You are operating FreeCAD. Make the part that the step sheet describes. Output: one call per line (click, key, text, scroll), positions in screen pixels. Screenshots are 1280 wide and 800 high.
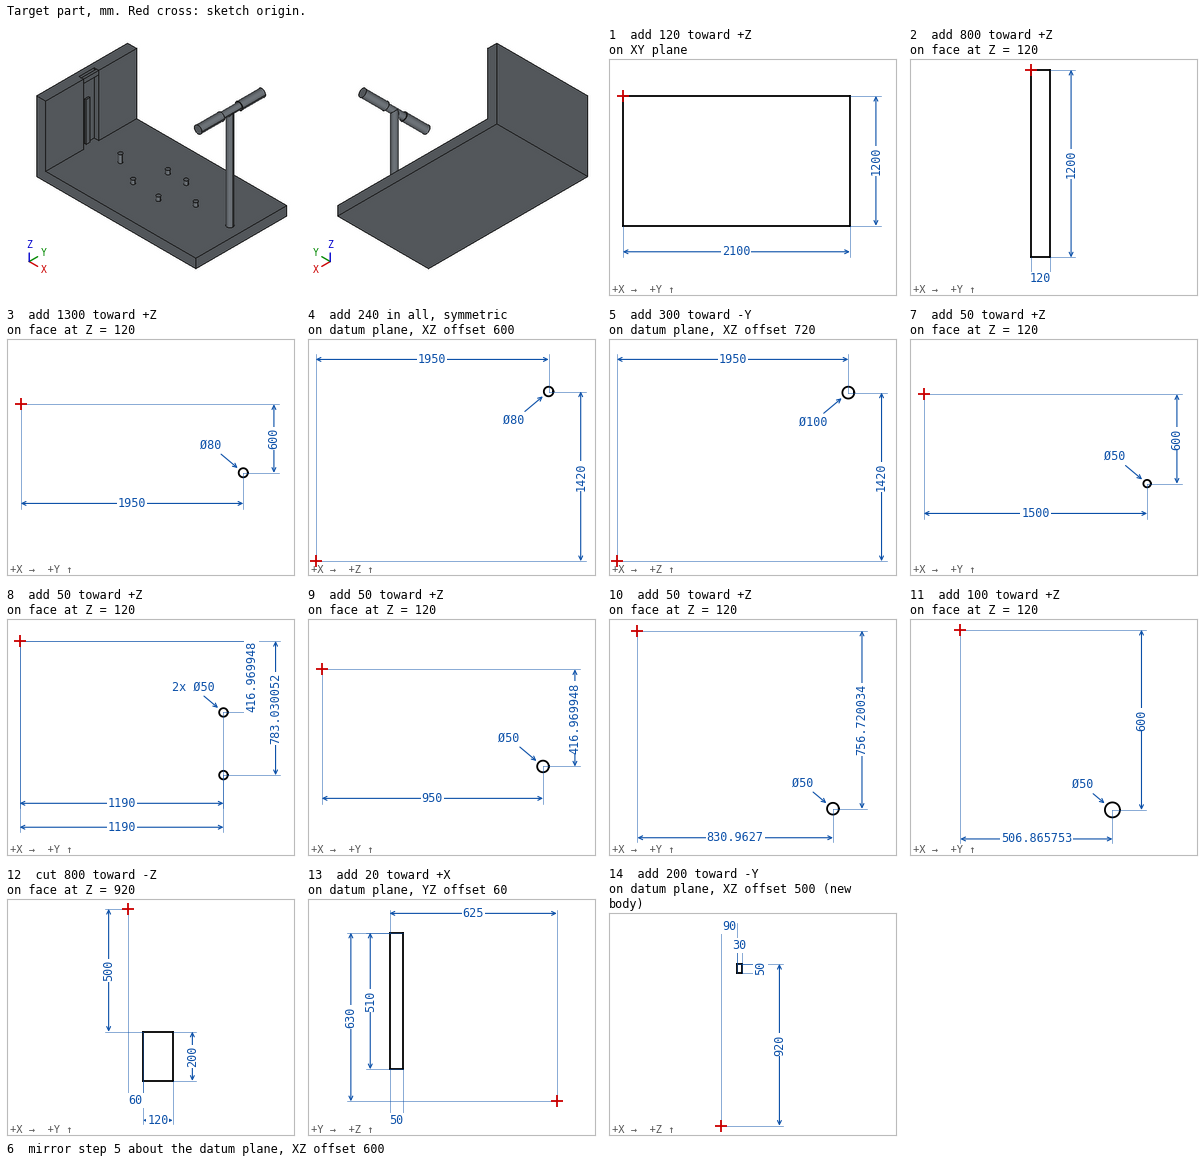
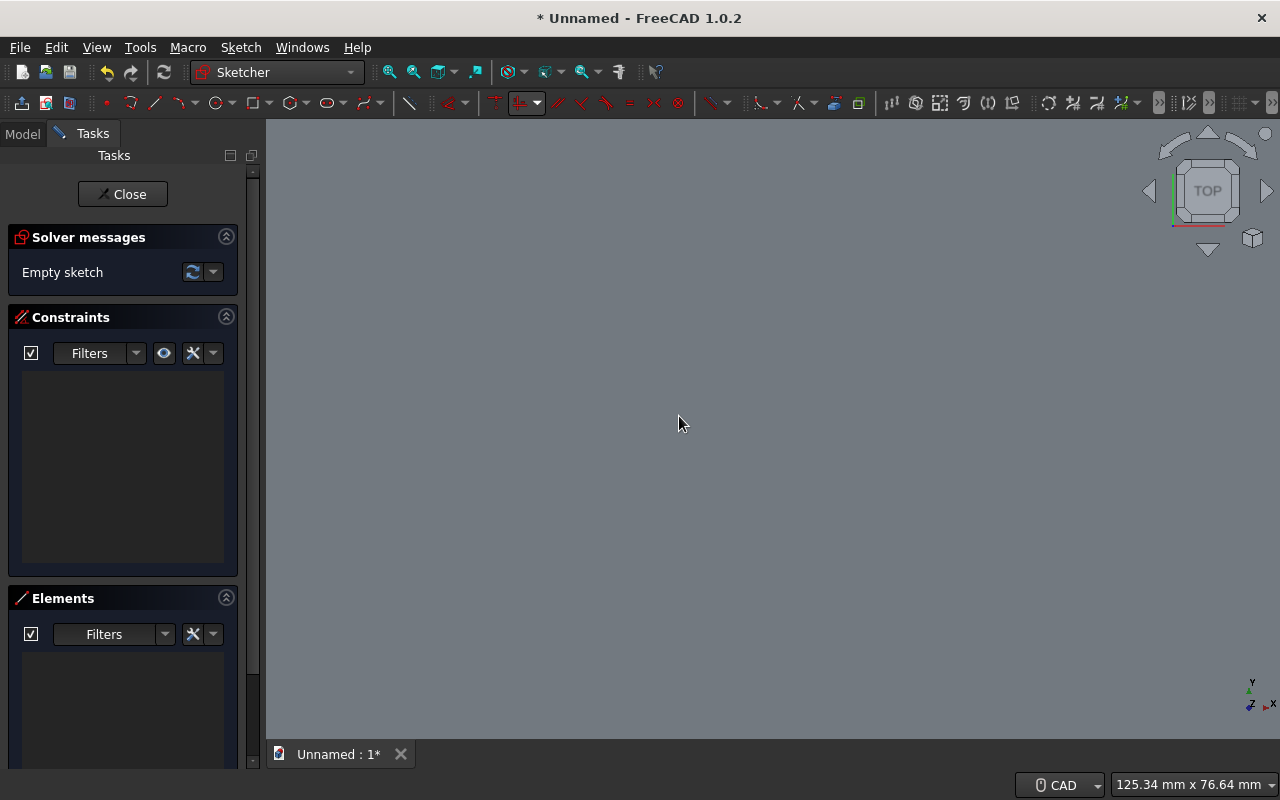
key(g)
key(c)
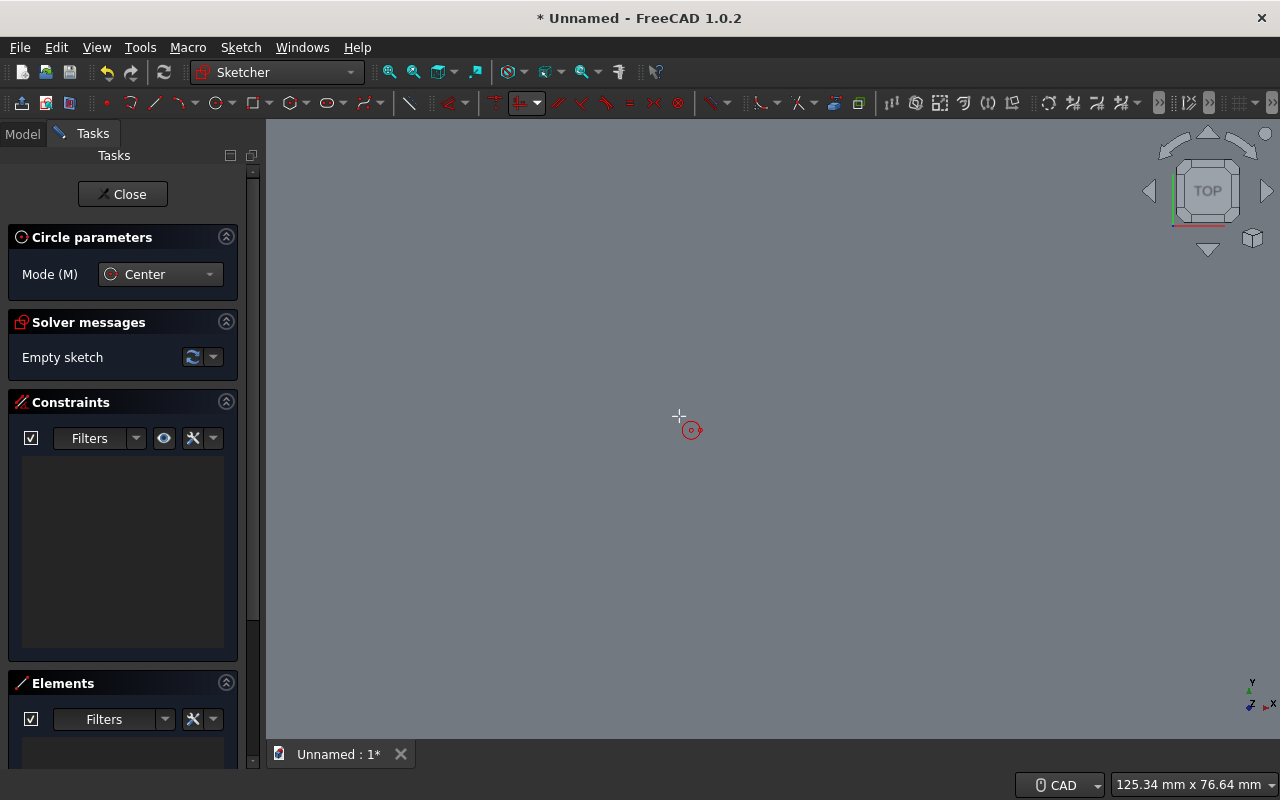
click(704, 429)
move(847, 285)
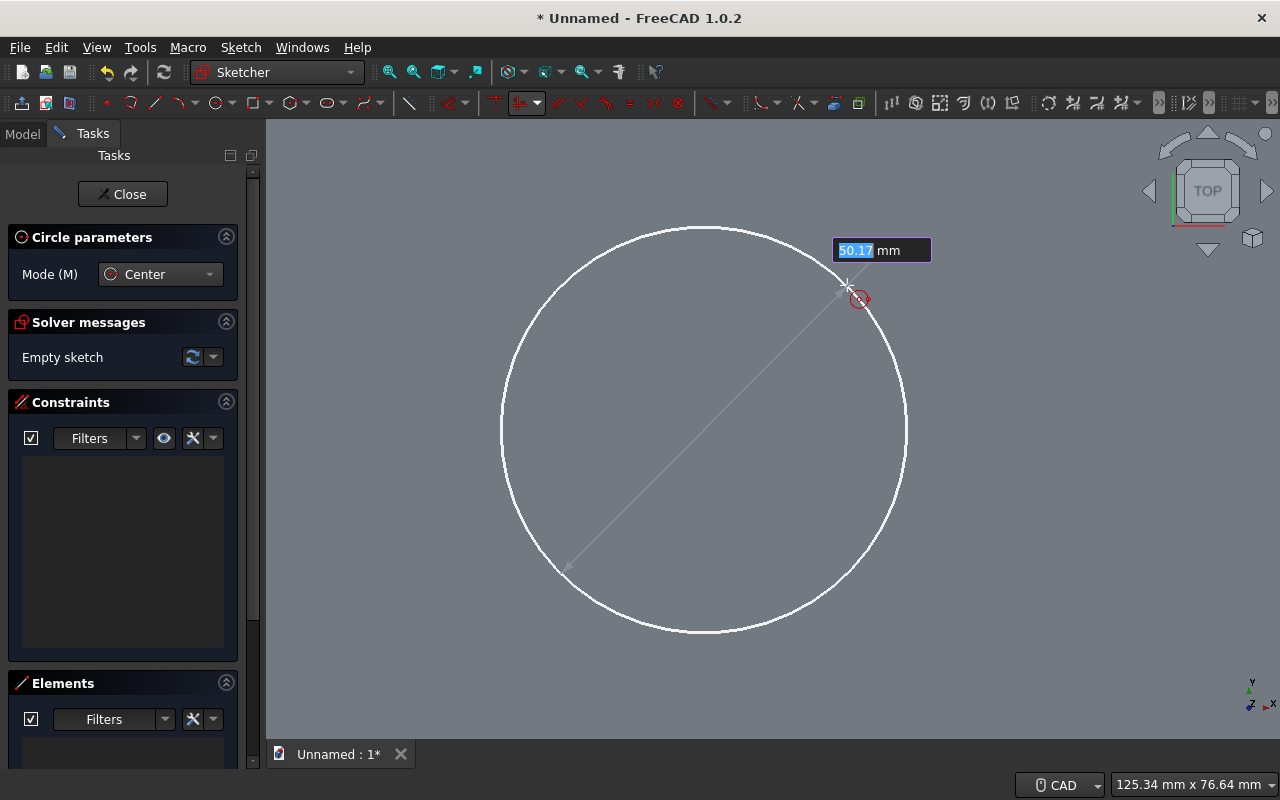
text(50)
key(Return)
key(Escape)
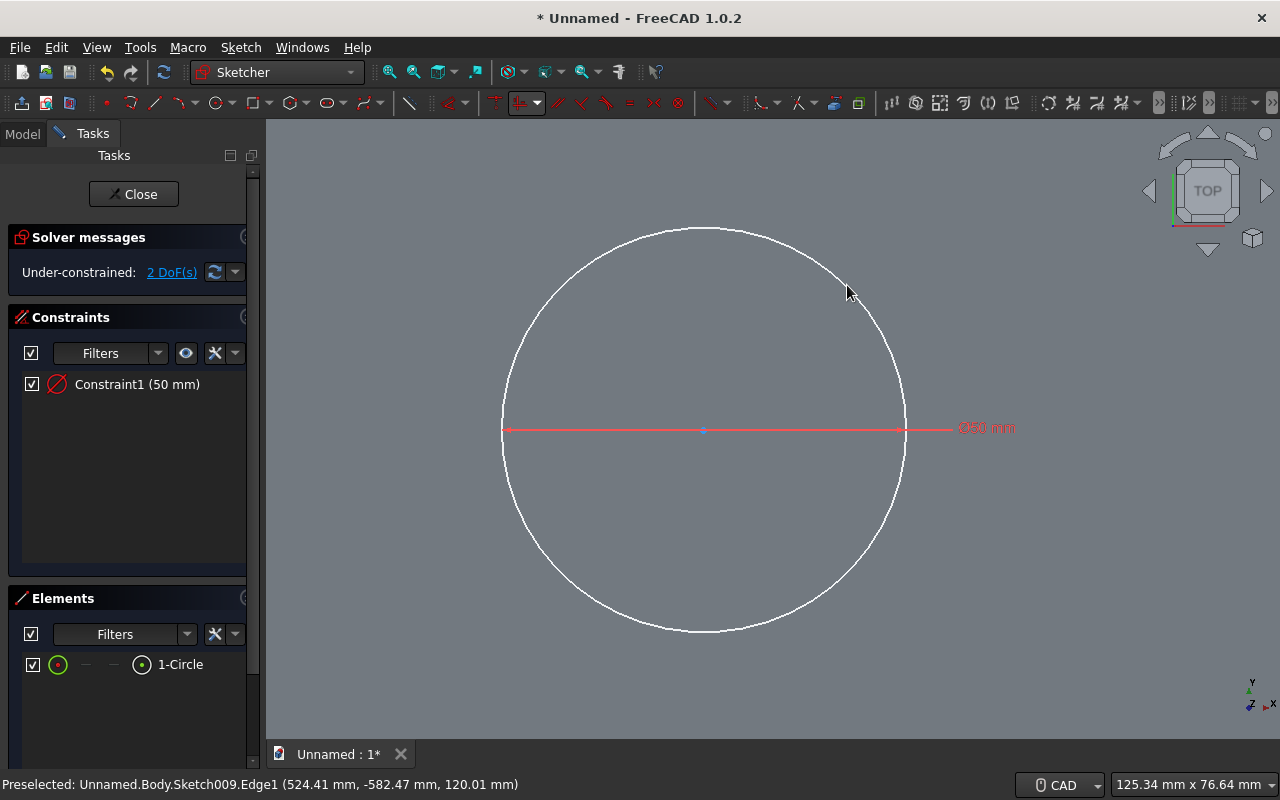
click(448, 104)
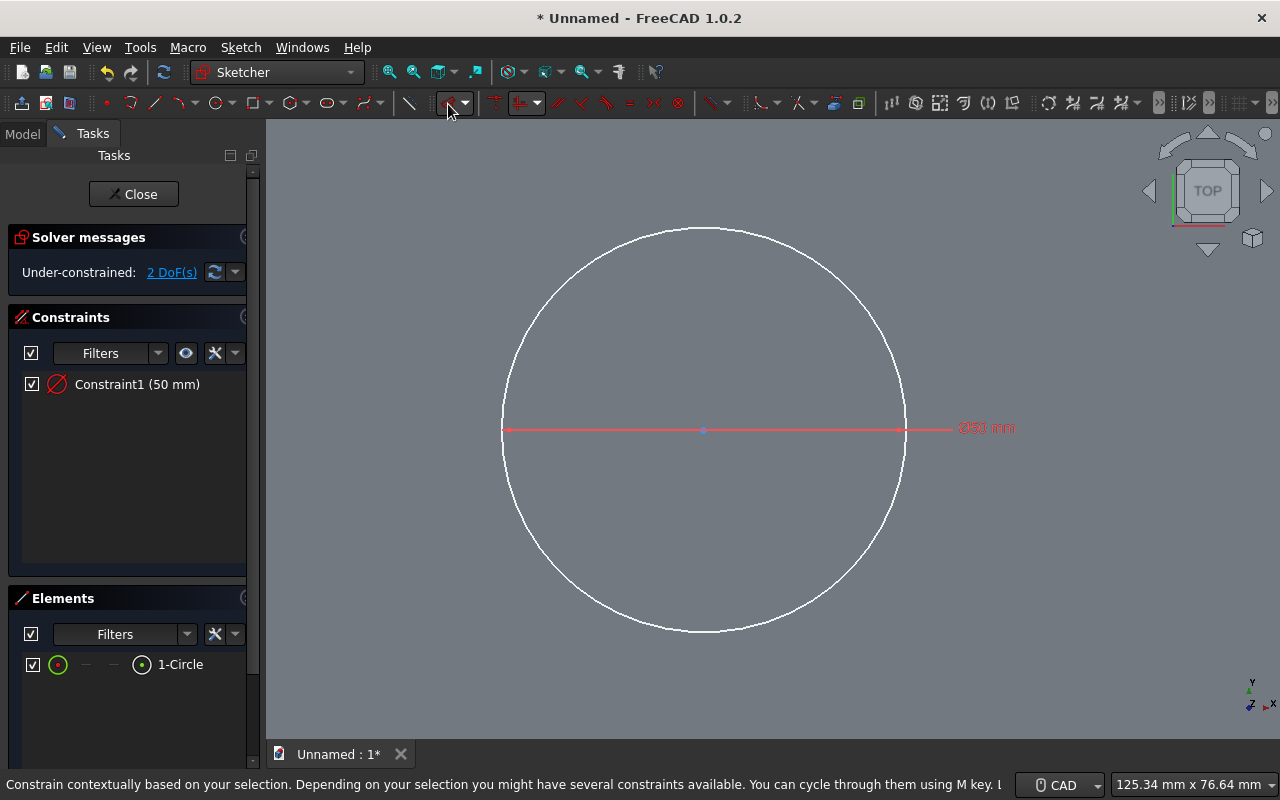
click(704, 430)
click(738, 288)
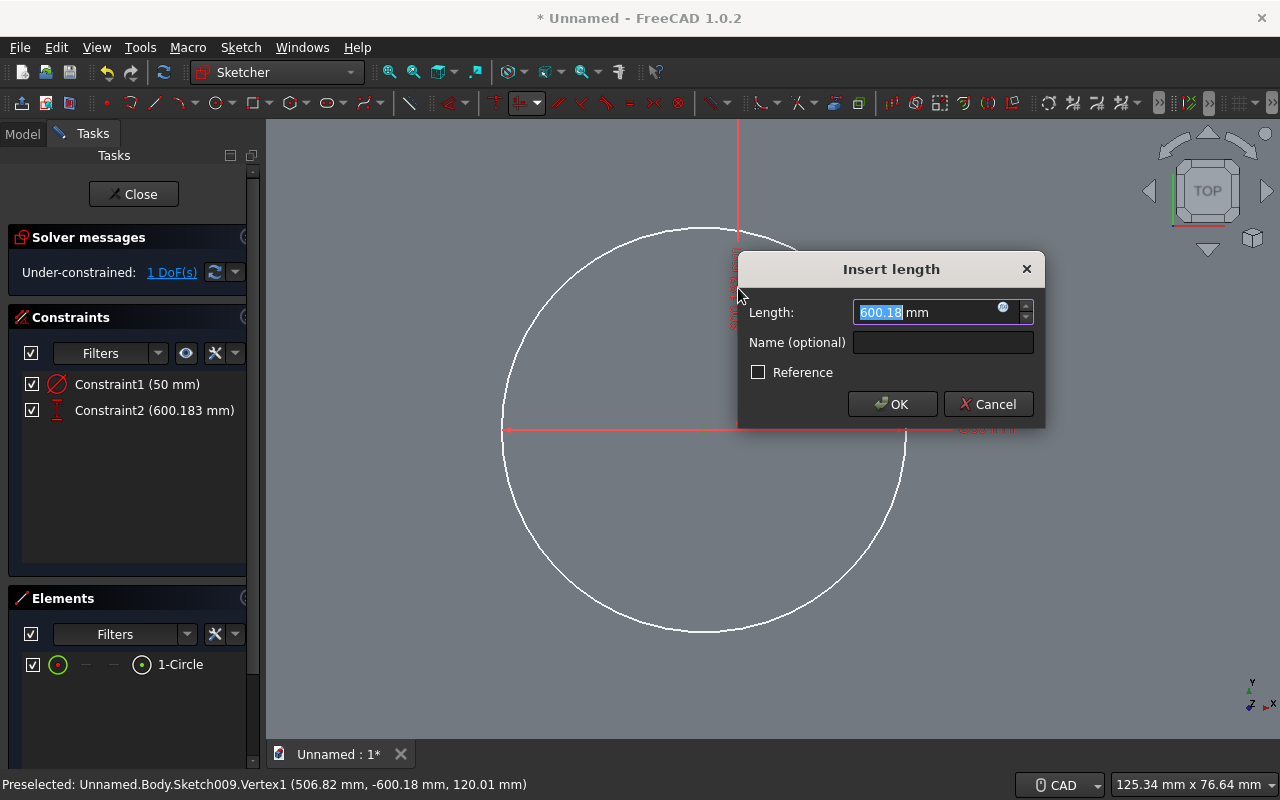
text(600)
key(Return)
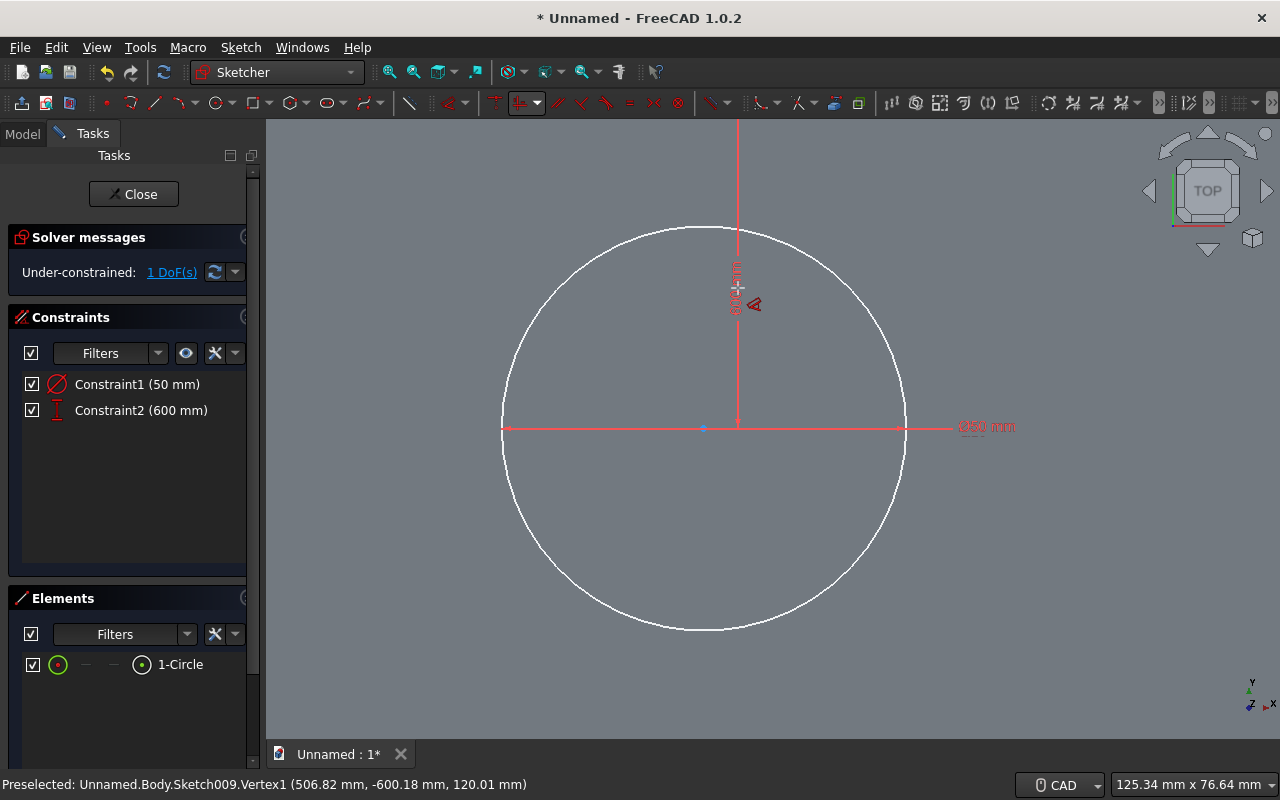
click(704, 429)
click(405, 463)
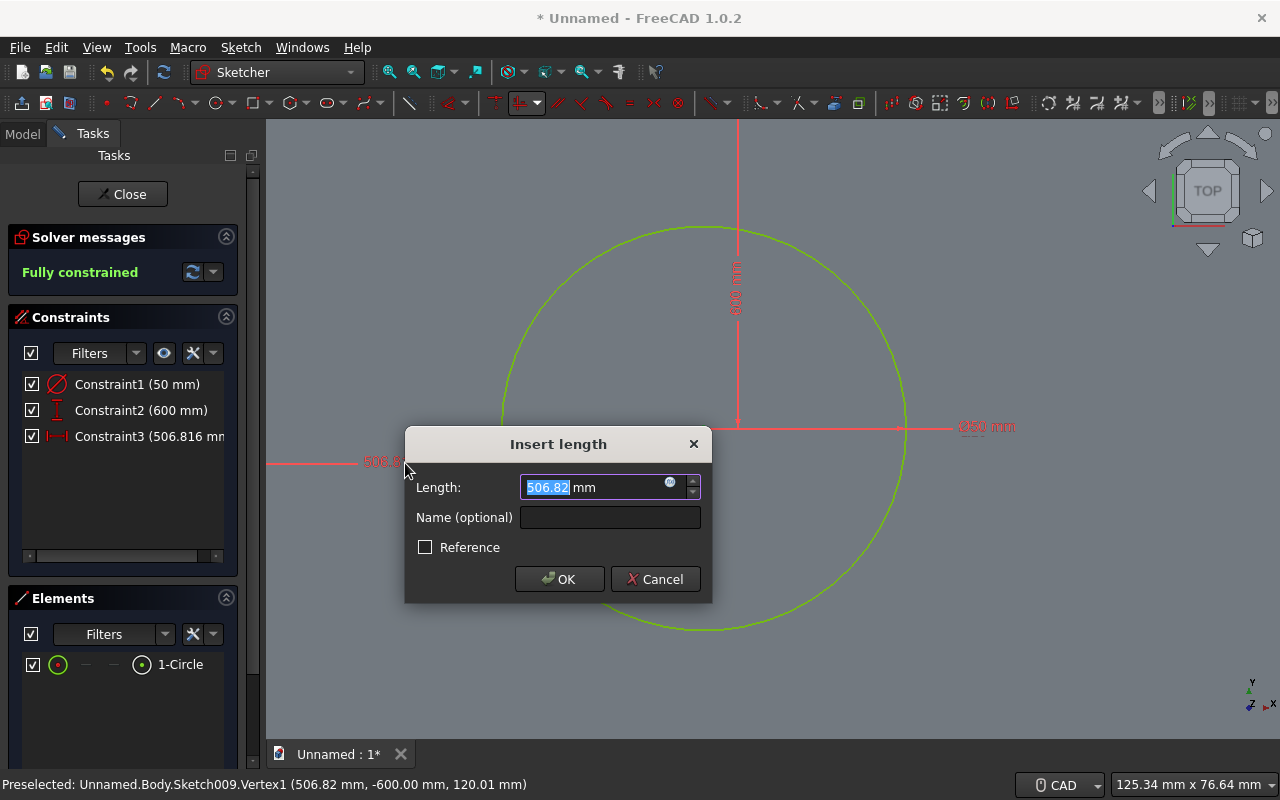
text(506.865753)
key(Return)
key(Escape)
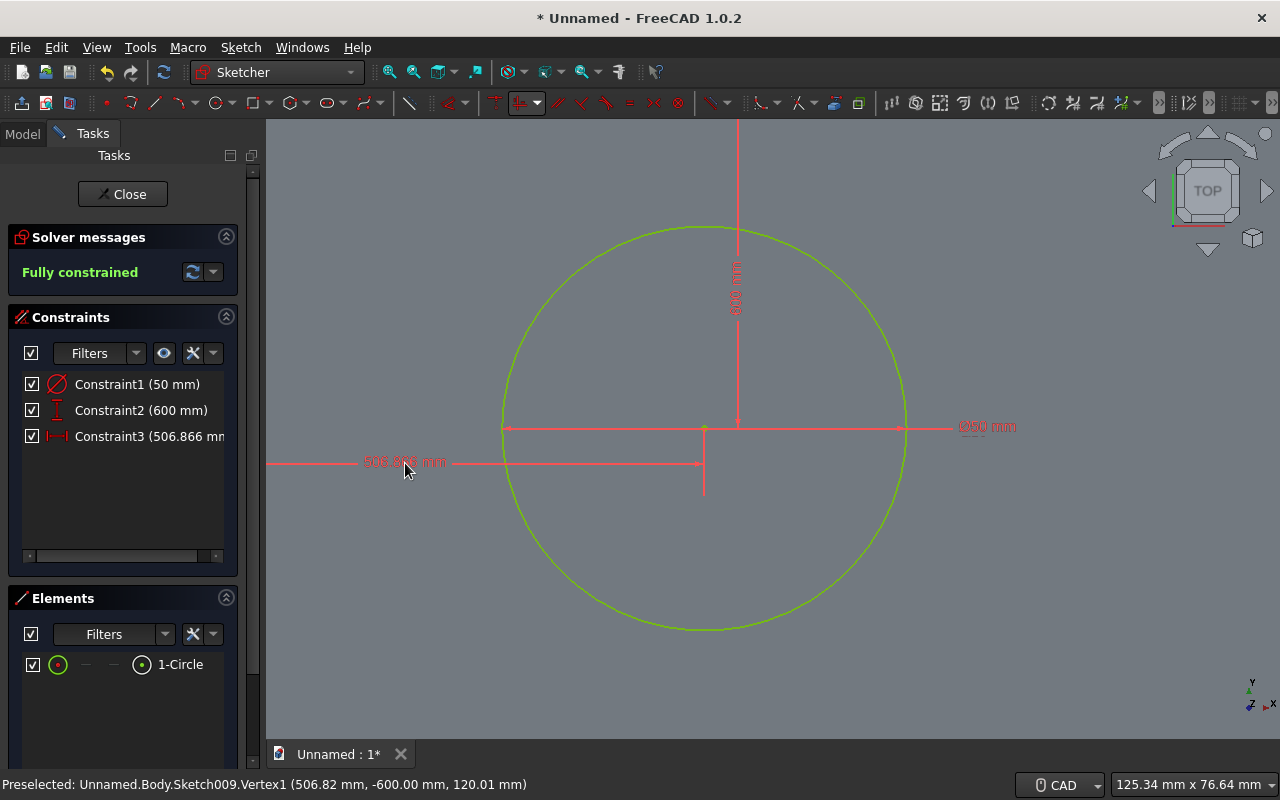
click(123, 194)